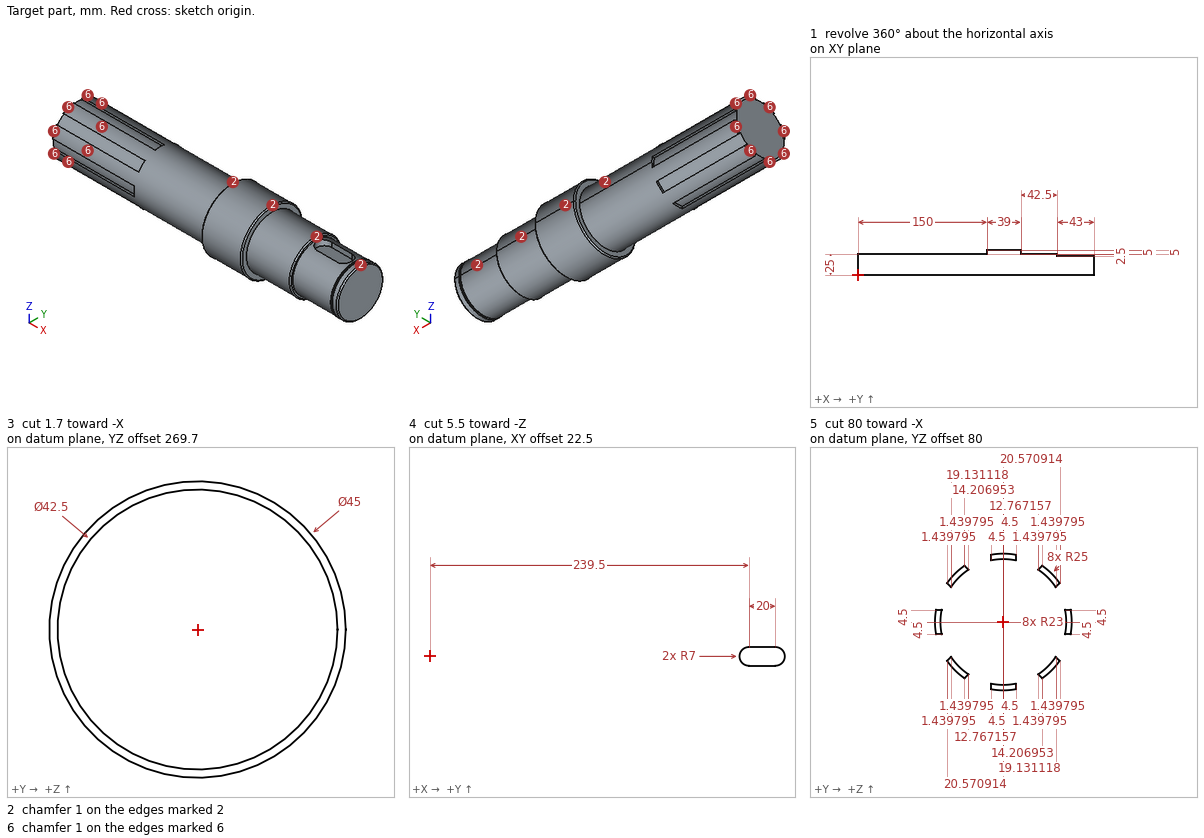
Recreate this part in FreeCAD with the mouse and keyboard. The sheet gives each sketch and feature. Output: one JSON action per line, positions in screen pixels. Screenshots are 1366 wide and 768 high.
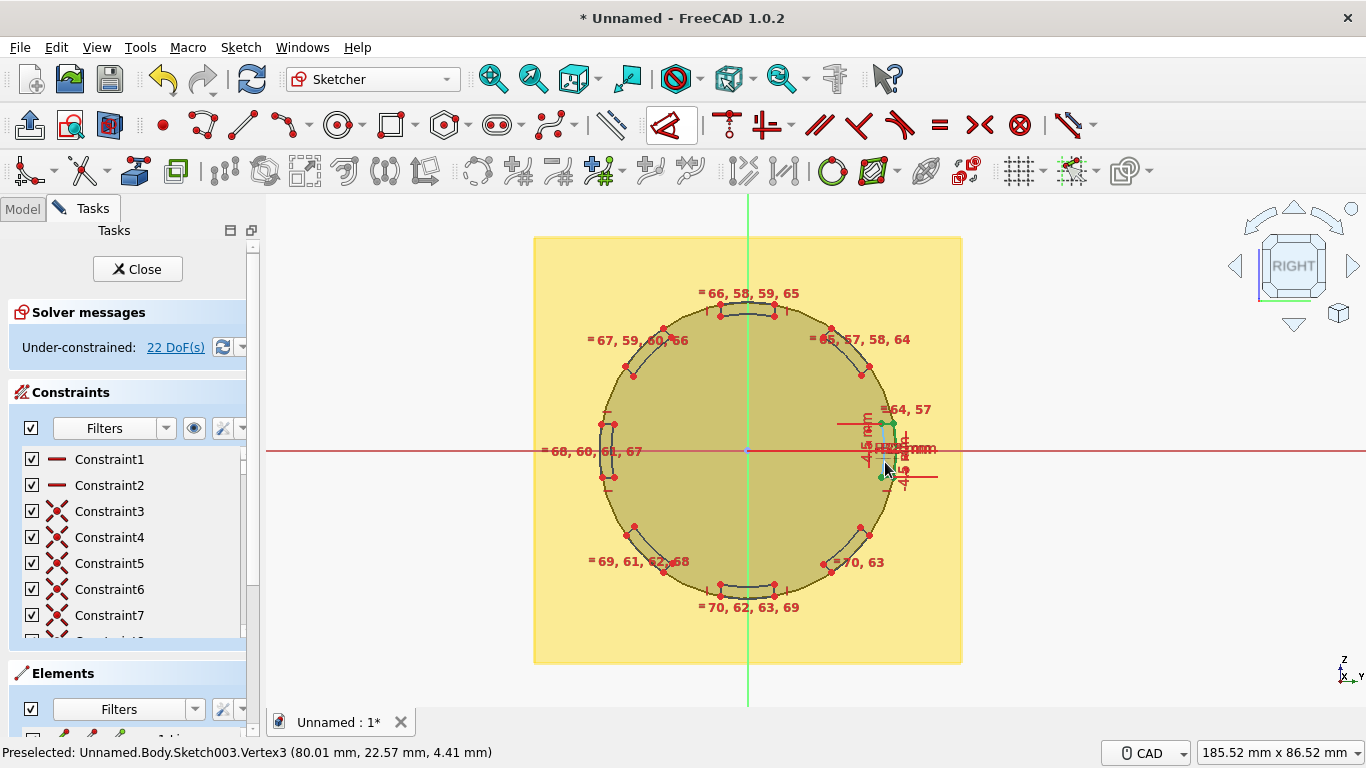
{"action": "scroll", "coordinate": [721, 317], "scroll_direction": "up", "scroll_amount": 2}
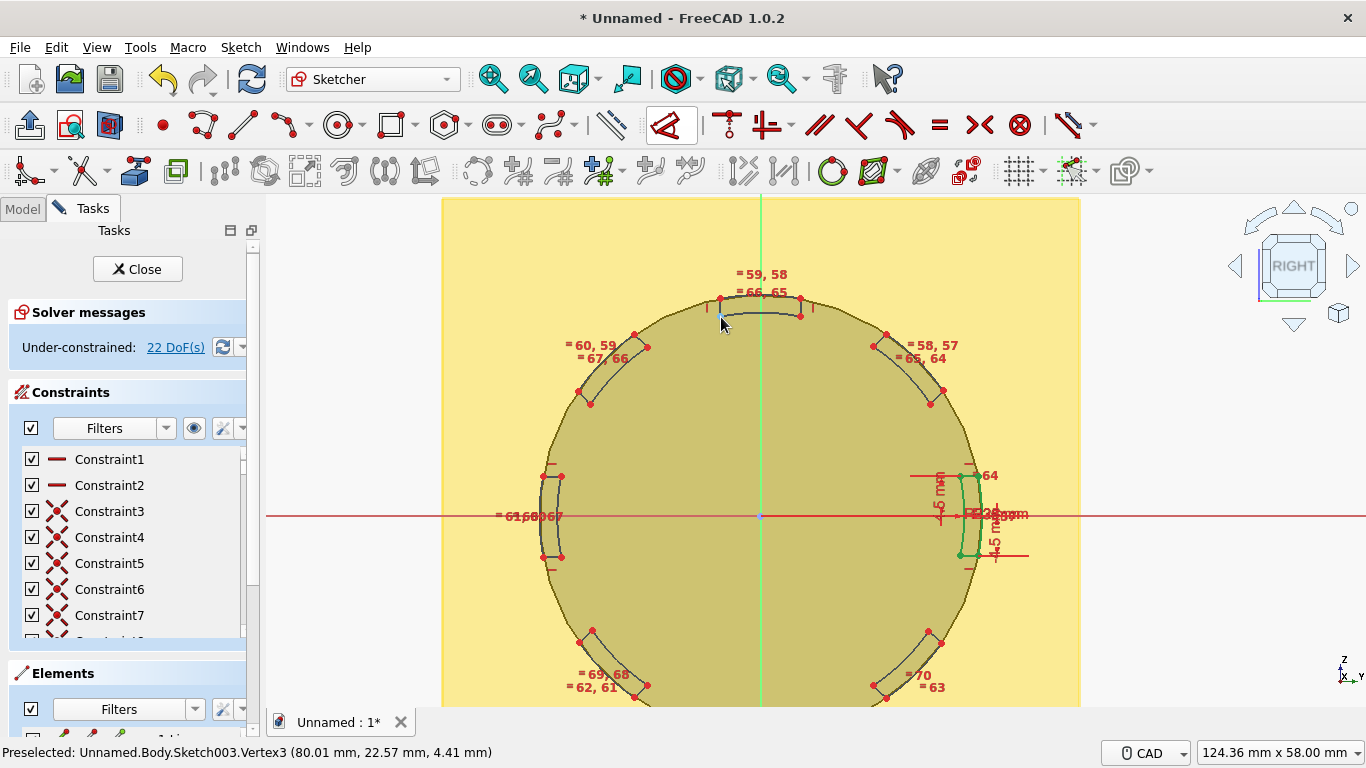
{"action": "left_click", "coordinate": [720, 317]}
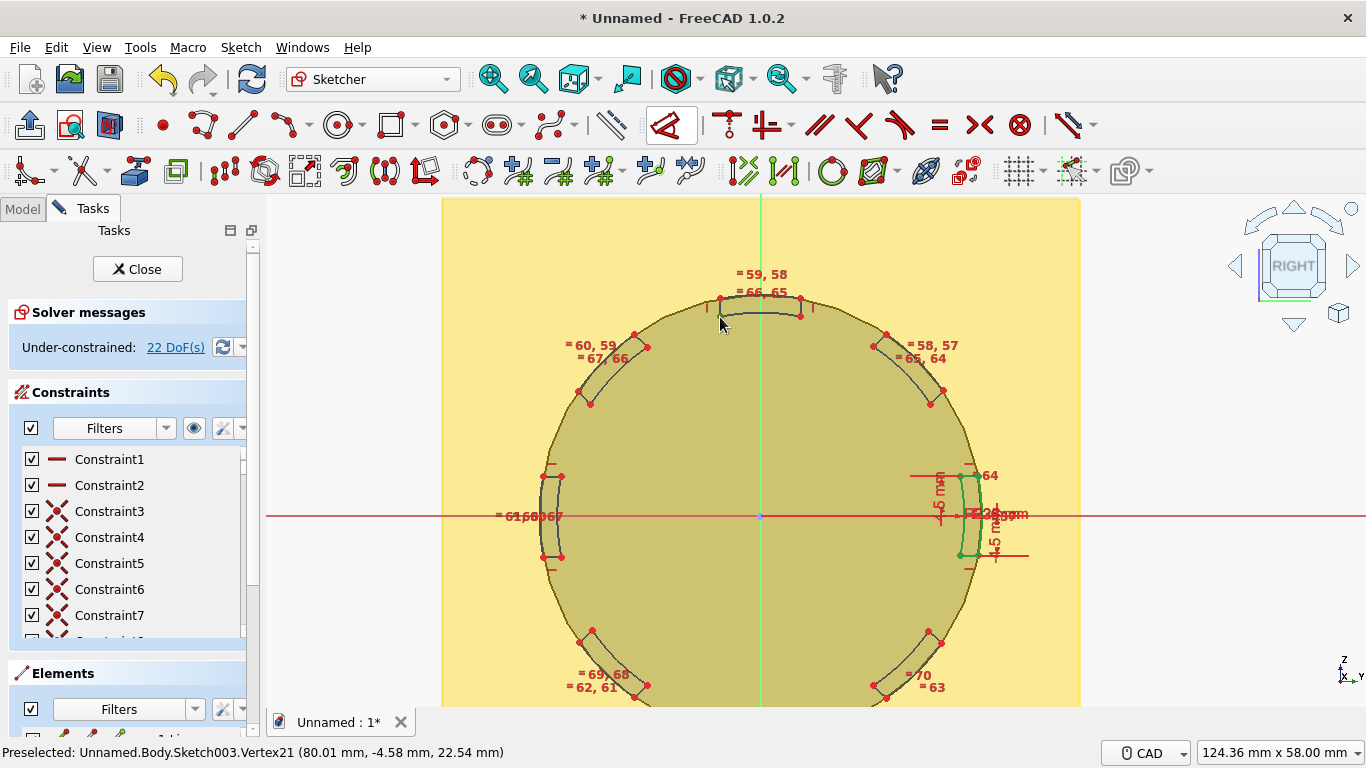
{"action": "left_click", "coordinate": [692, 126]}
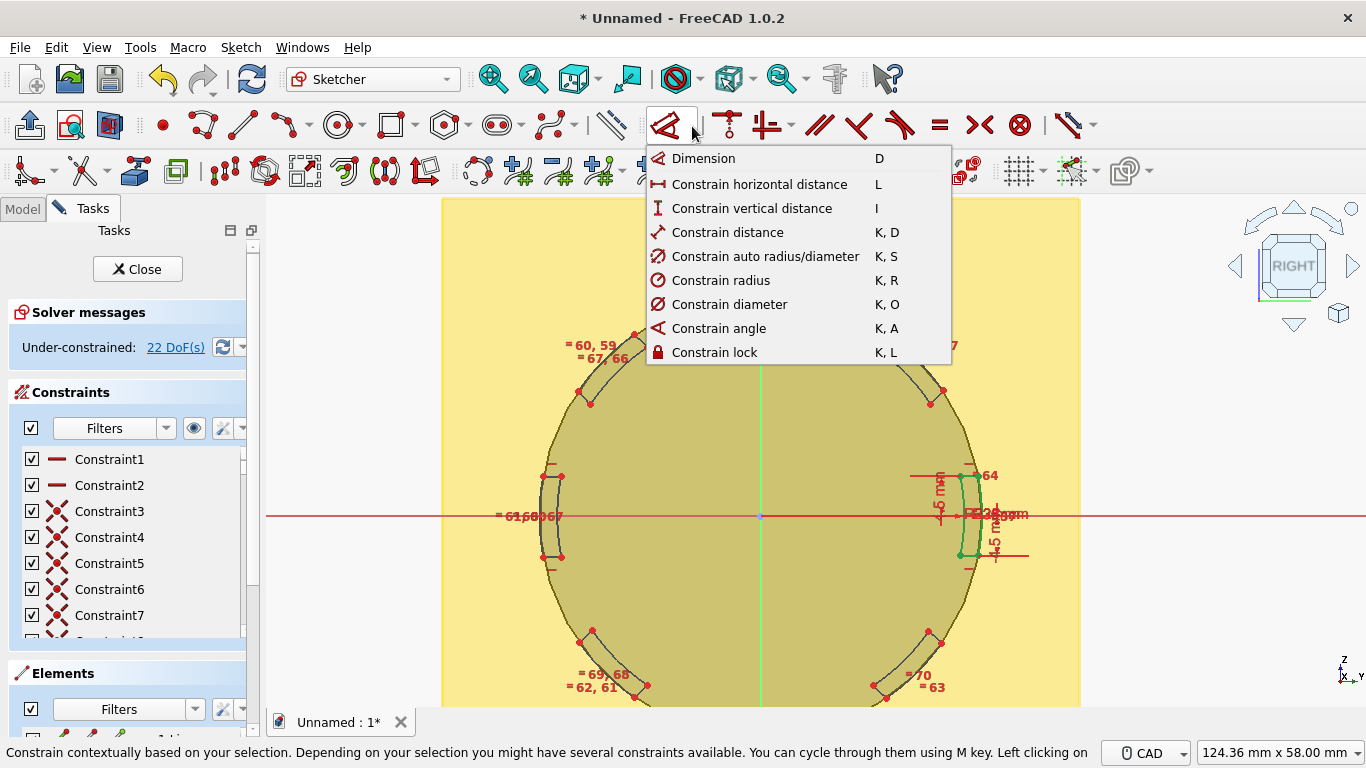
{"action": "left_click", "coordinate": [799, 184]}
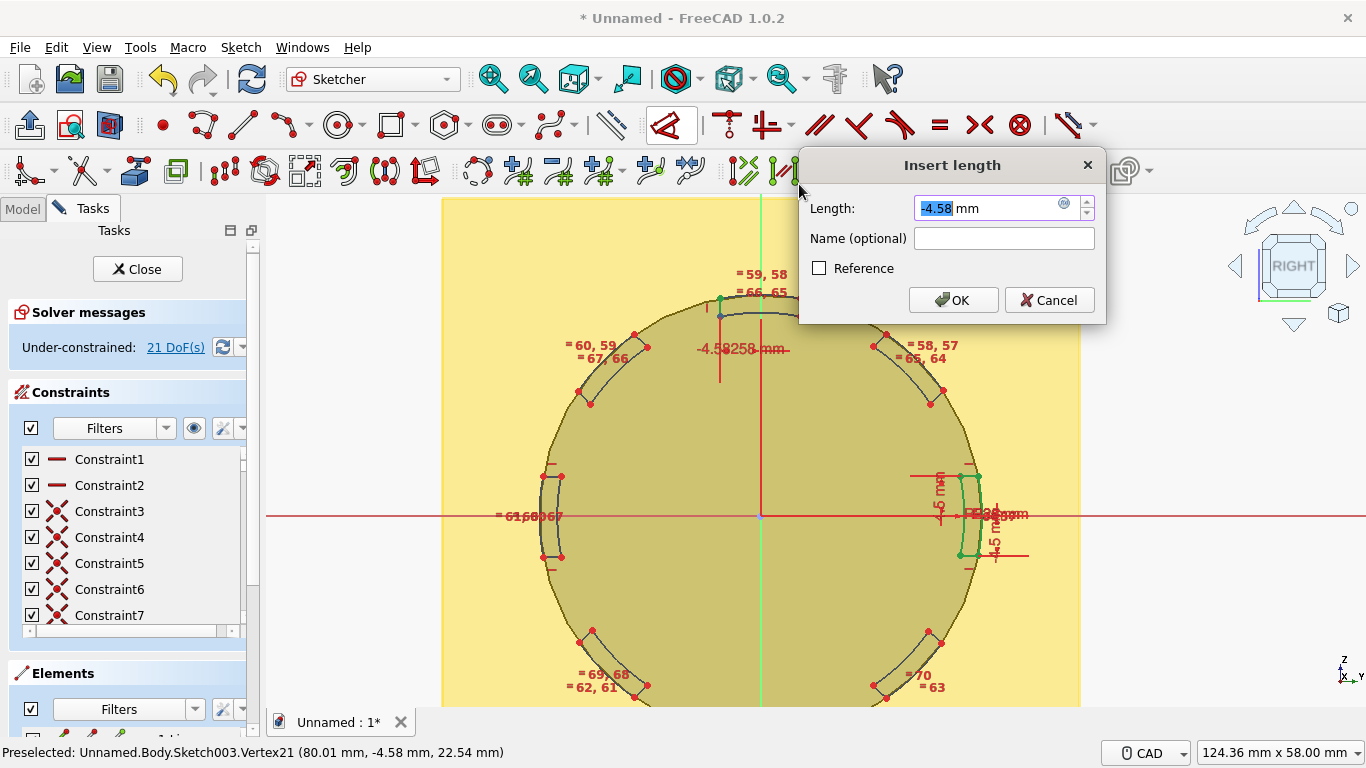
{"action": "type", "text": "-4.5"}
{"action": "key", "text": "Return"}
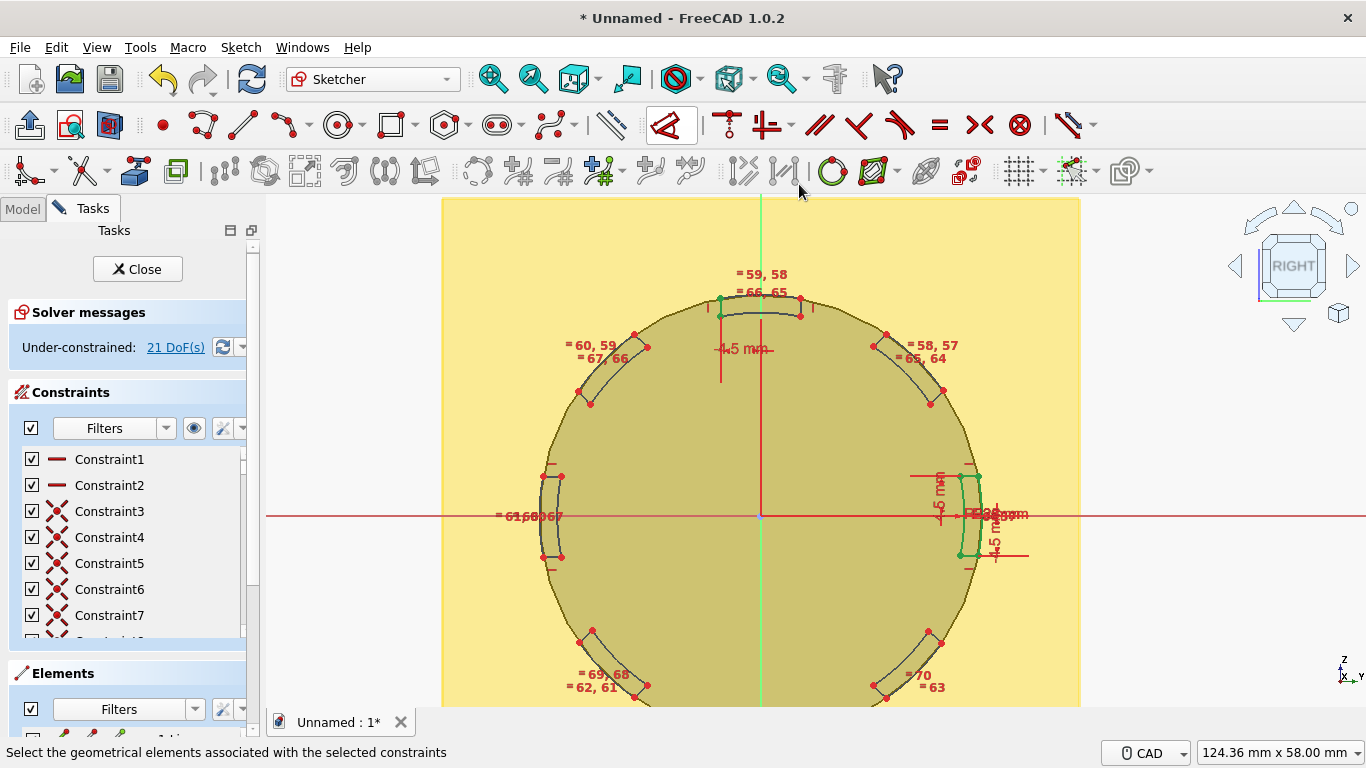
{"action": "left_click", "coordinate": [801, 299]}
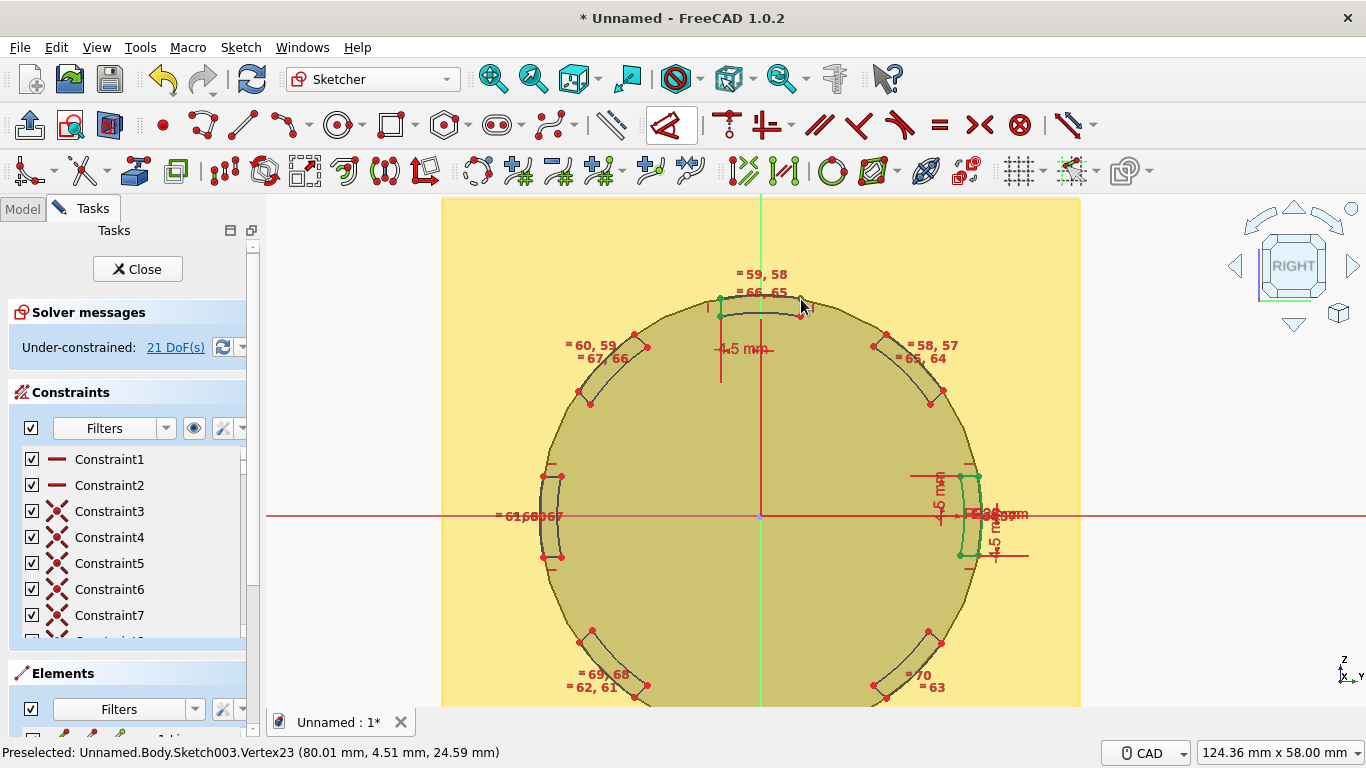
{"action": "key", "text": "l"}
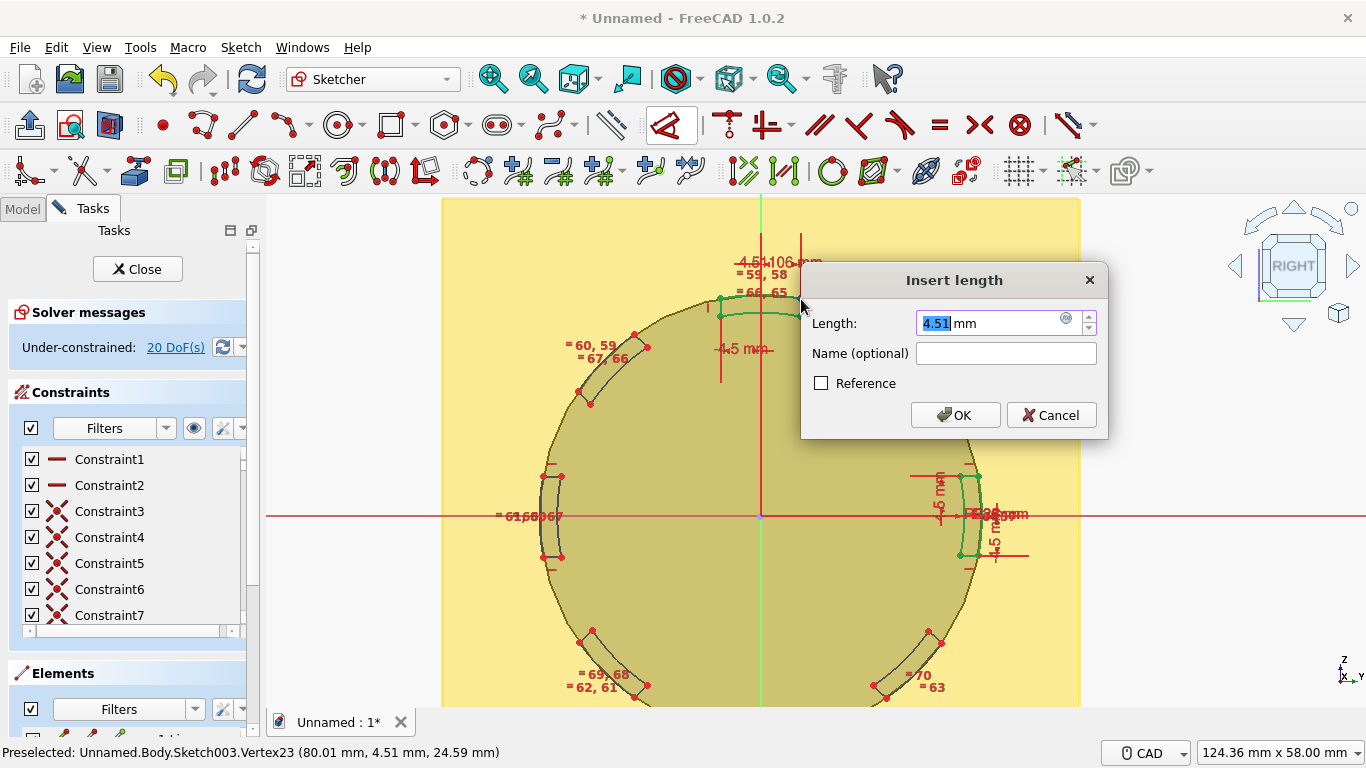
{"action": "type", "text": "4.5"}
{"action": "key", "text": "Return"}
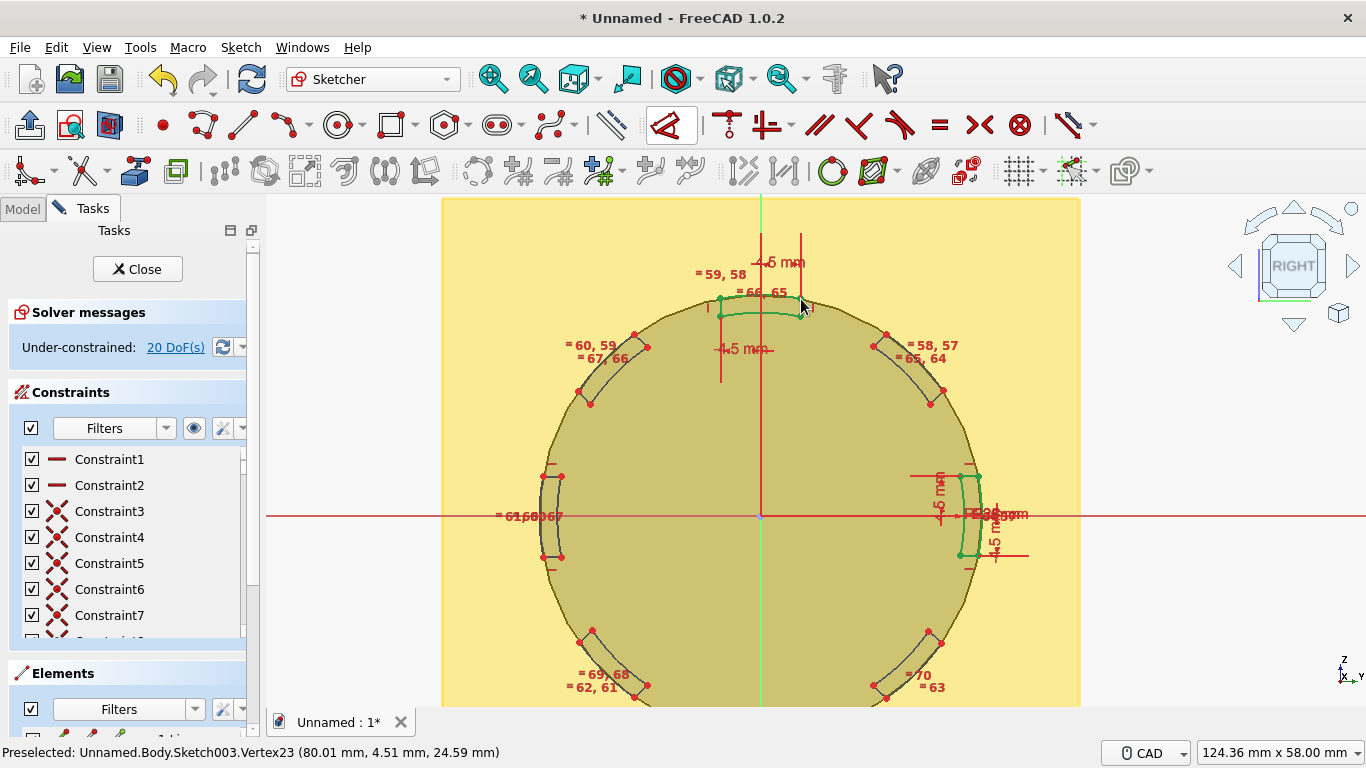
{"action": "left_click", "coordinate": [561, 557]}